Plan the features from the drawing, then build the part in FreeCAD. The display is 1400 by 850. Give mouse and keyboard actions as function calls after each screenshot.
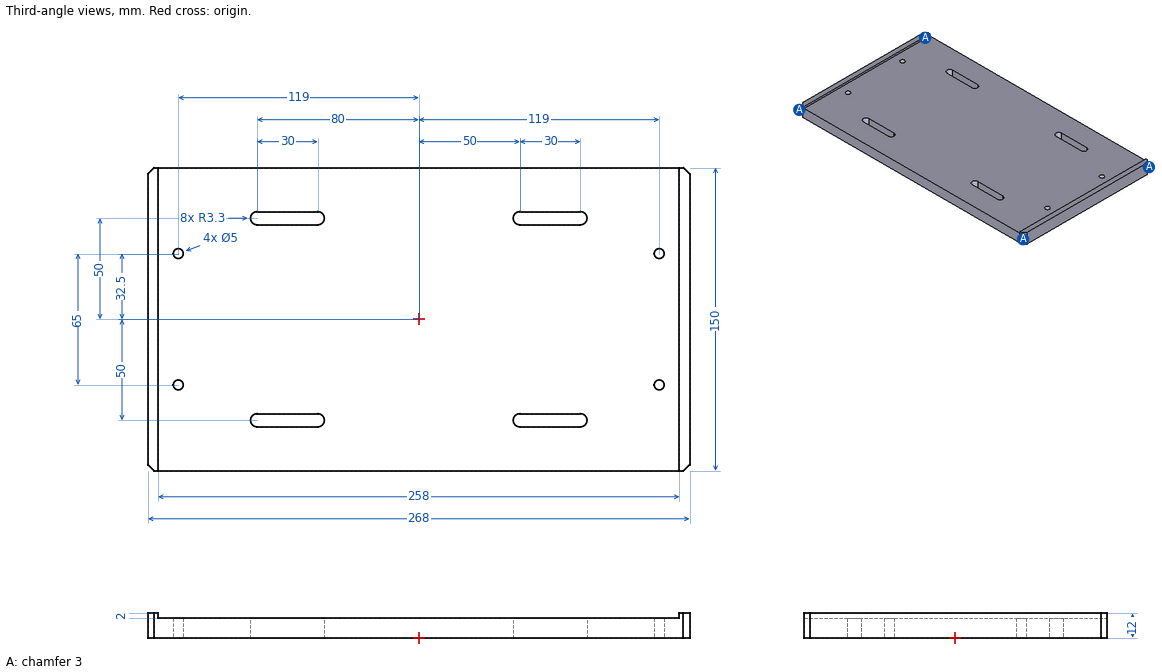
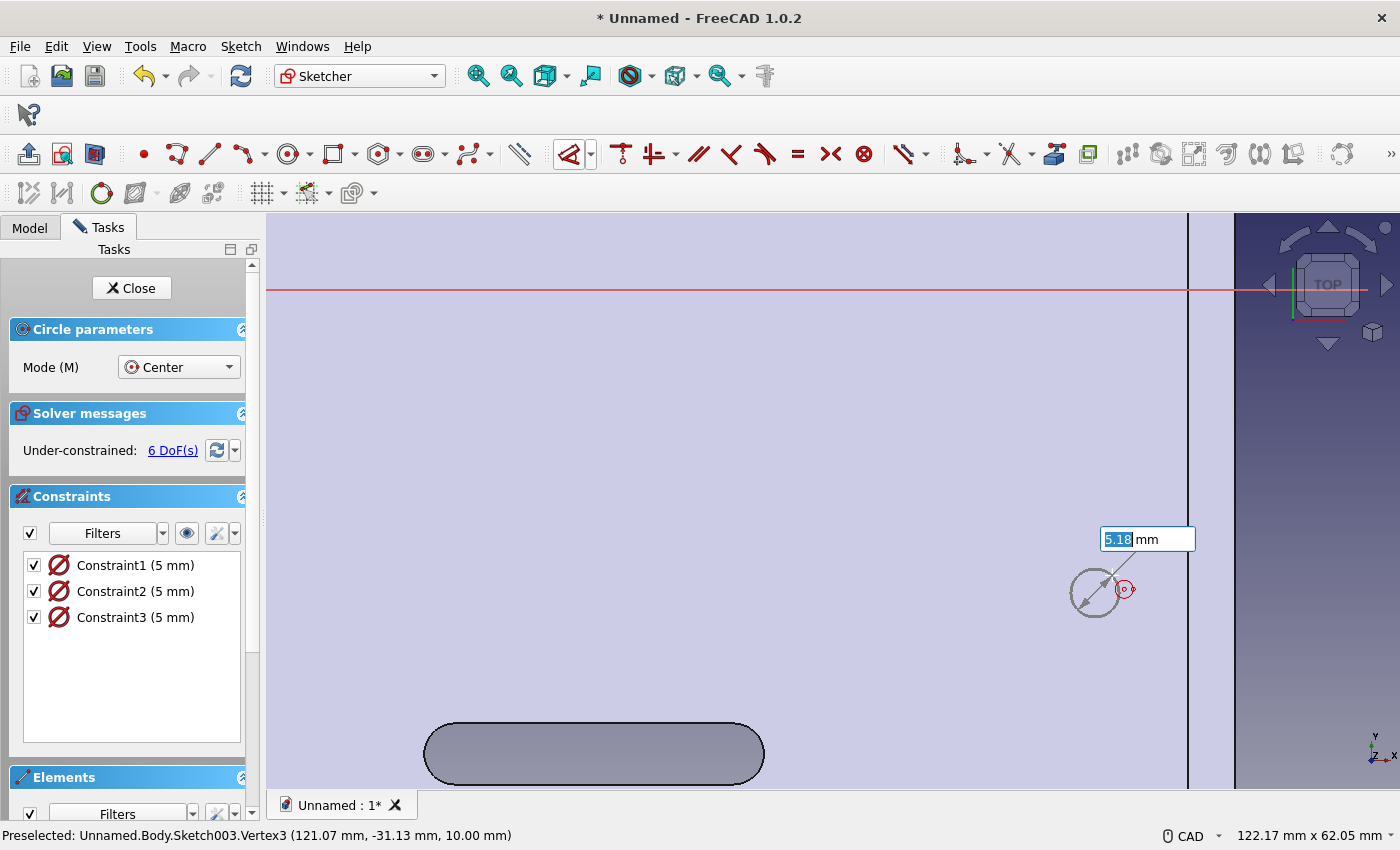
text(5)
key(Return)
key(Escape)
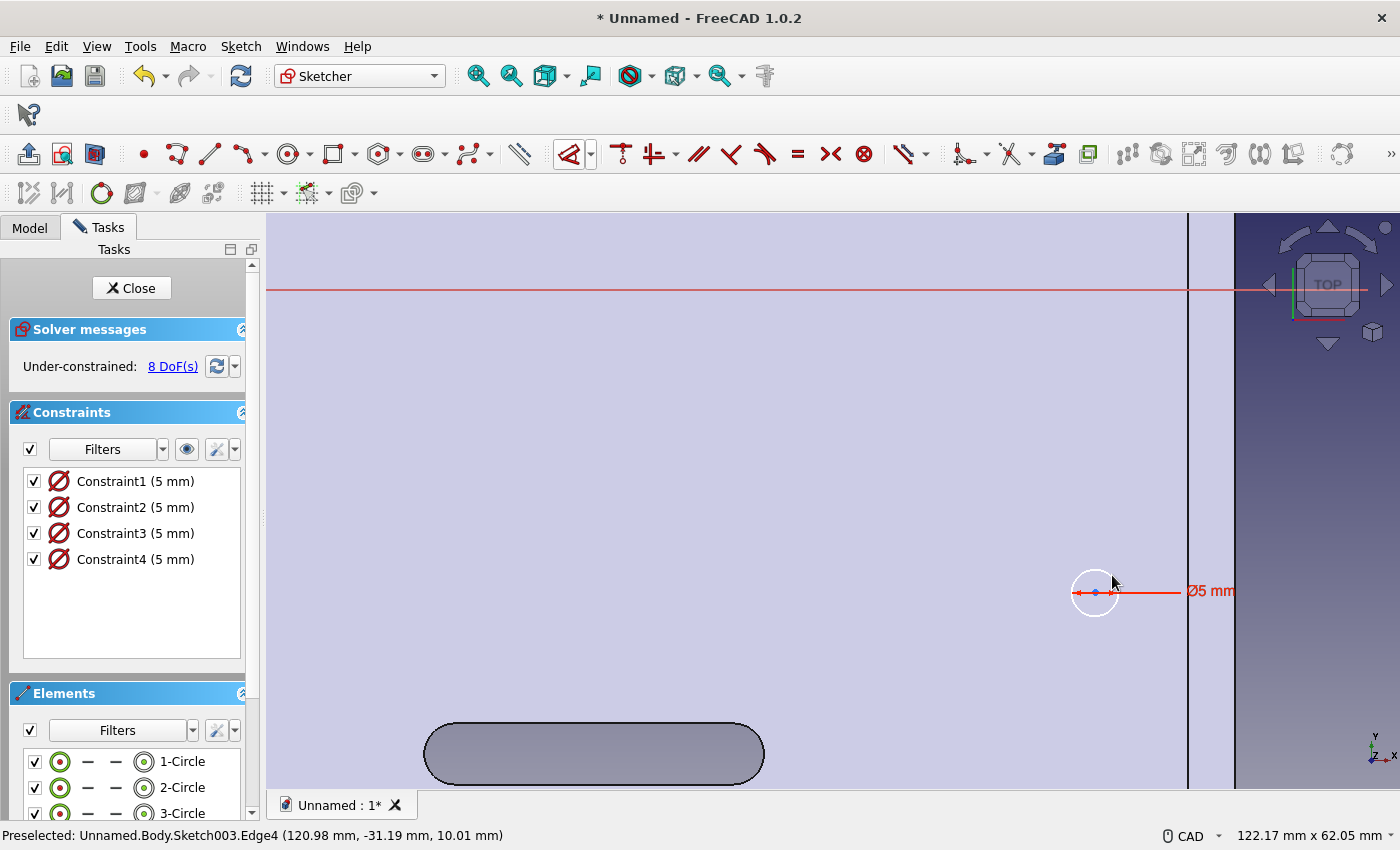
scroll(1098, 592, down, 6)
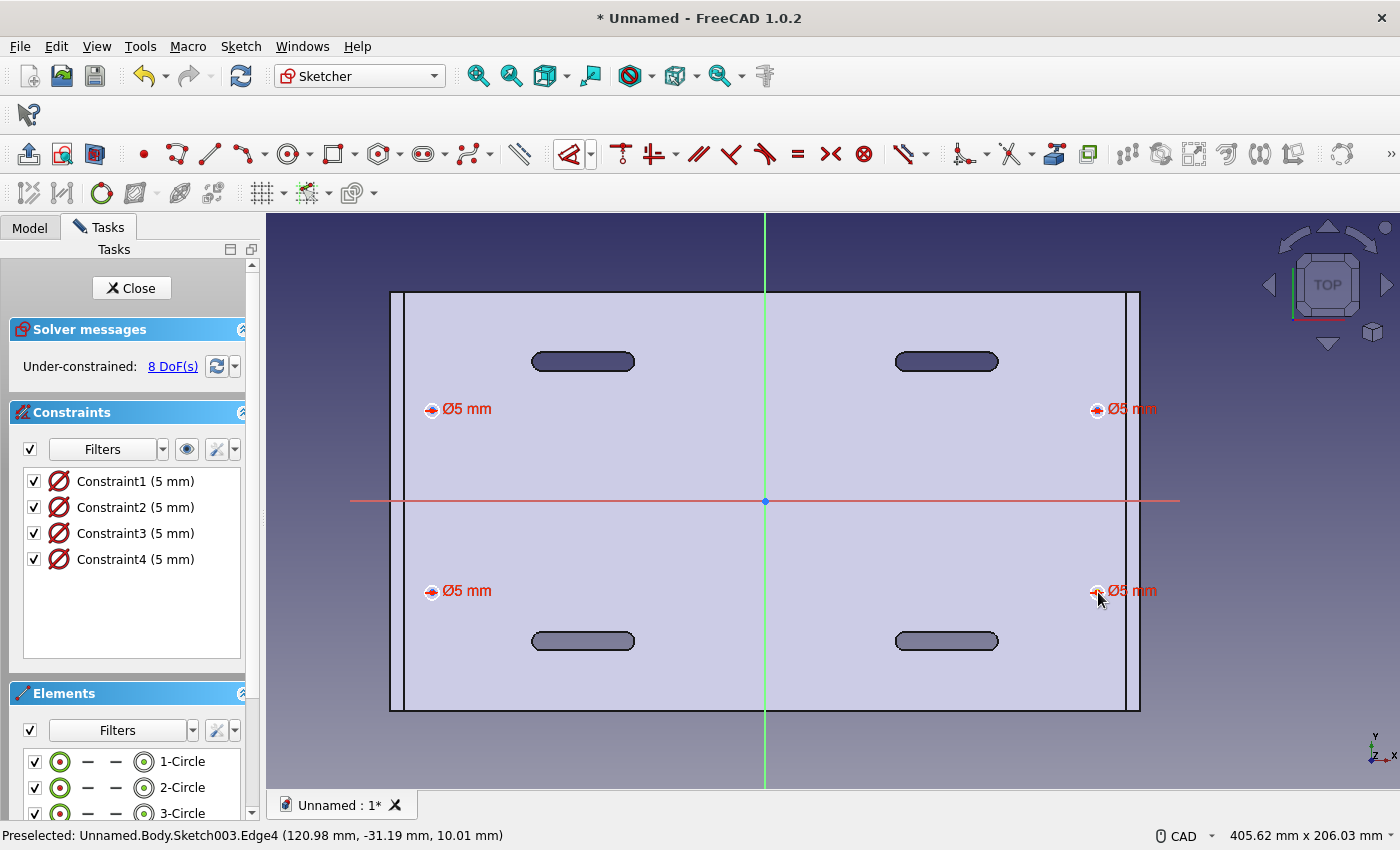
click(432, 411)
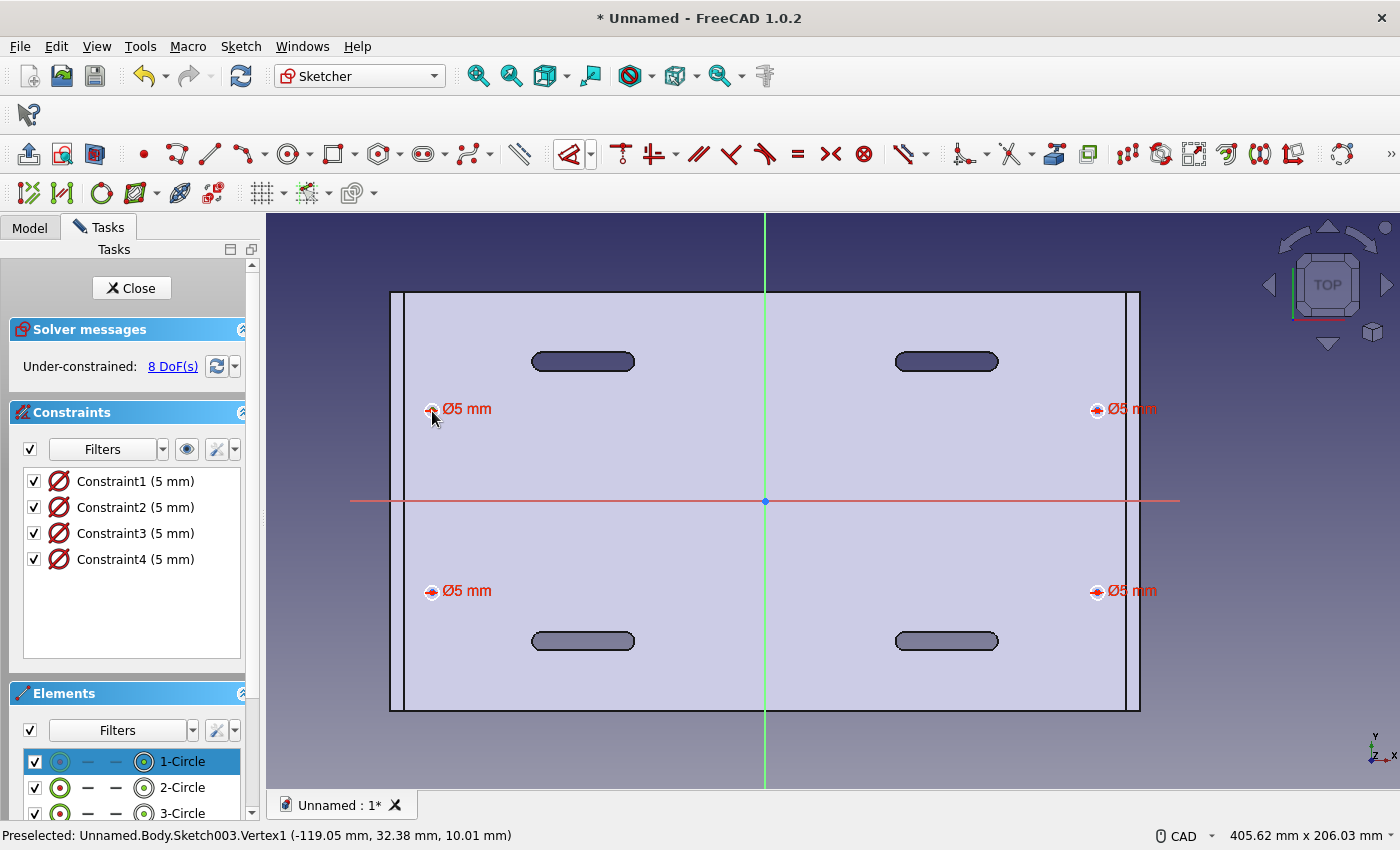
click(432, 593)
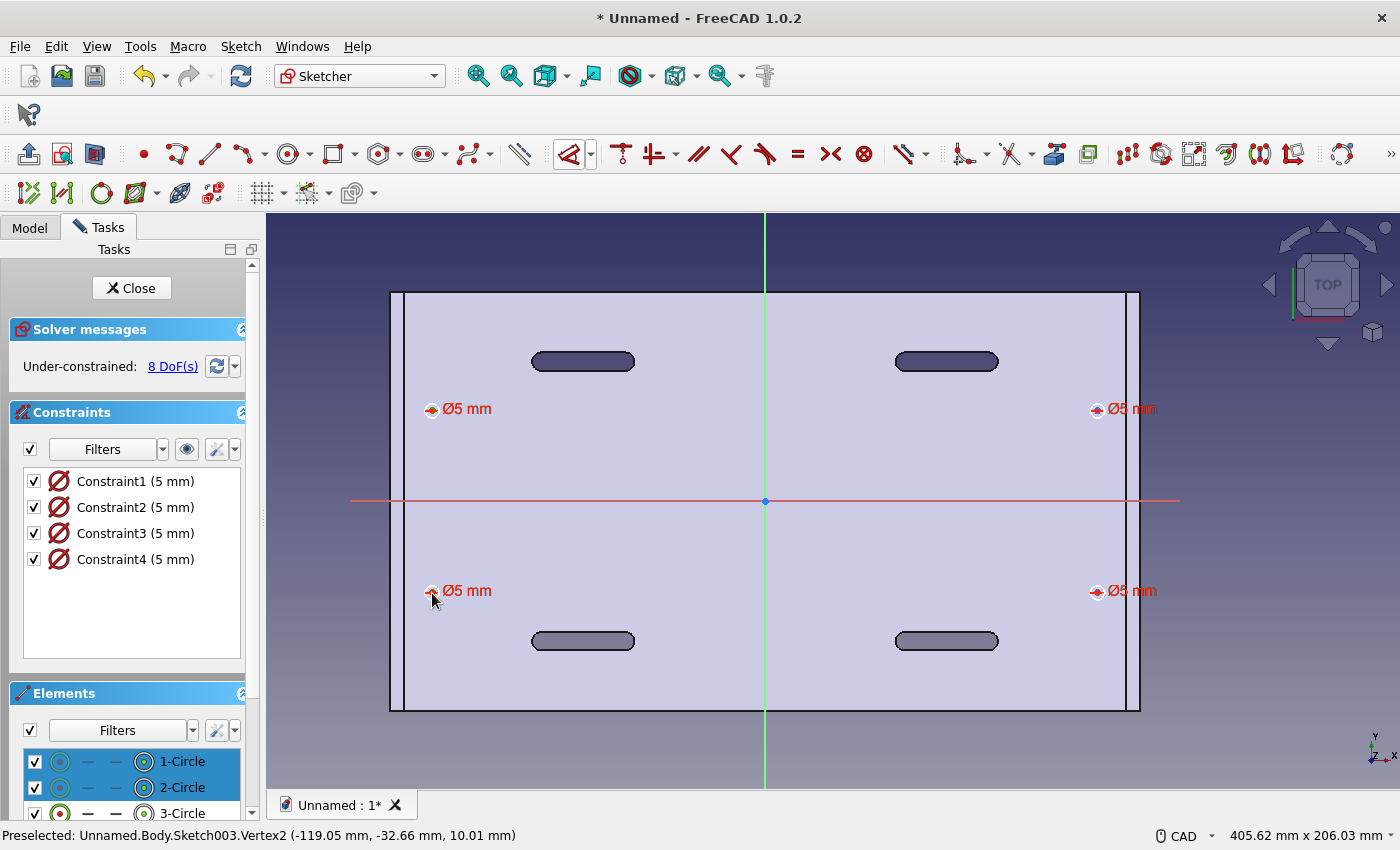
click(676, 154)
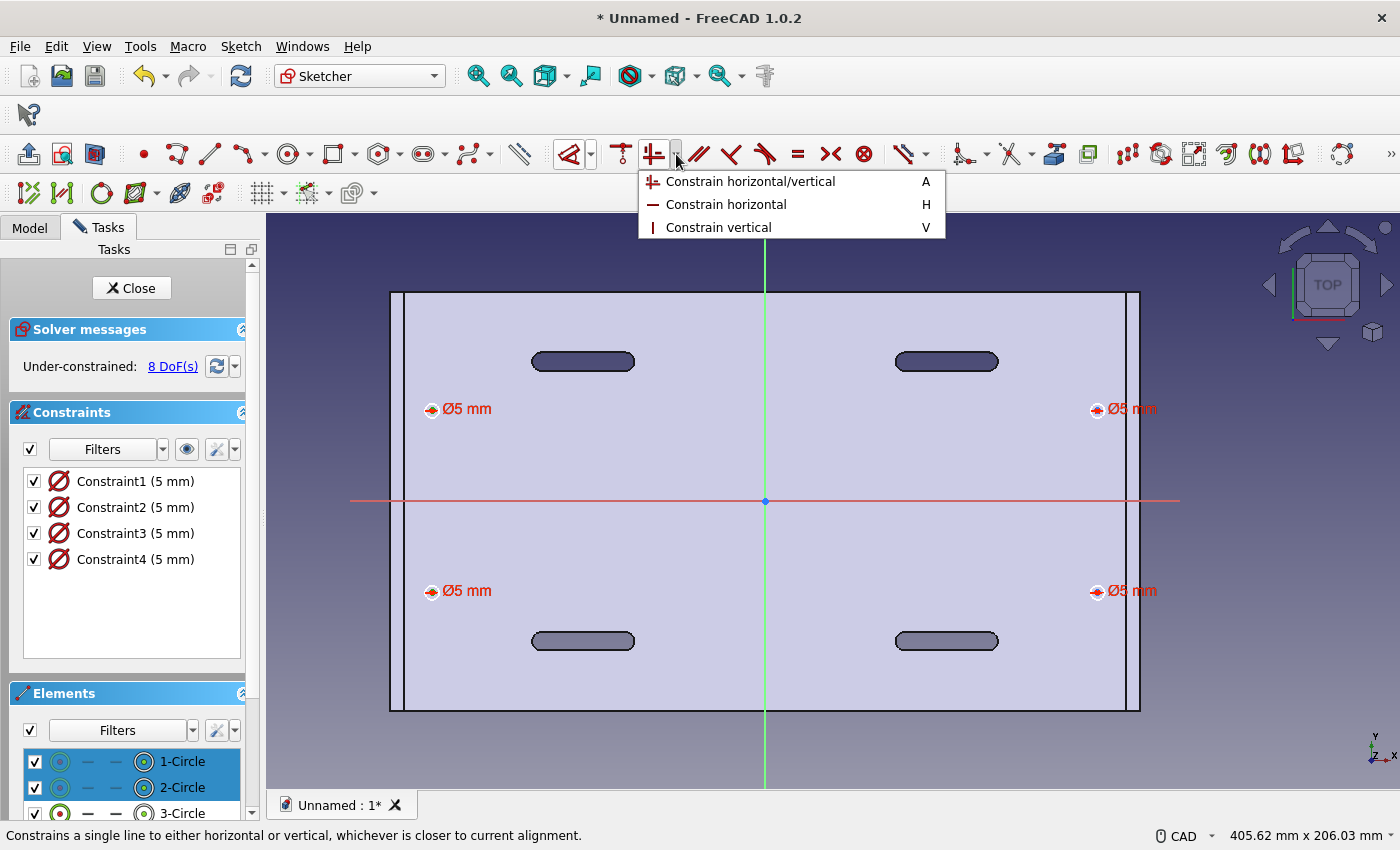
click(792, 228)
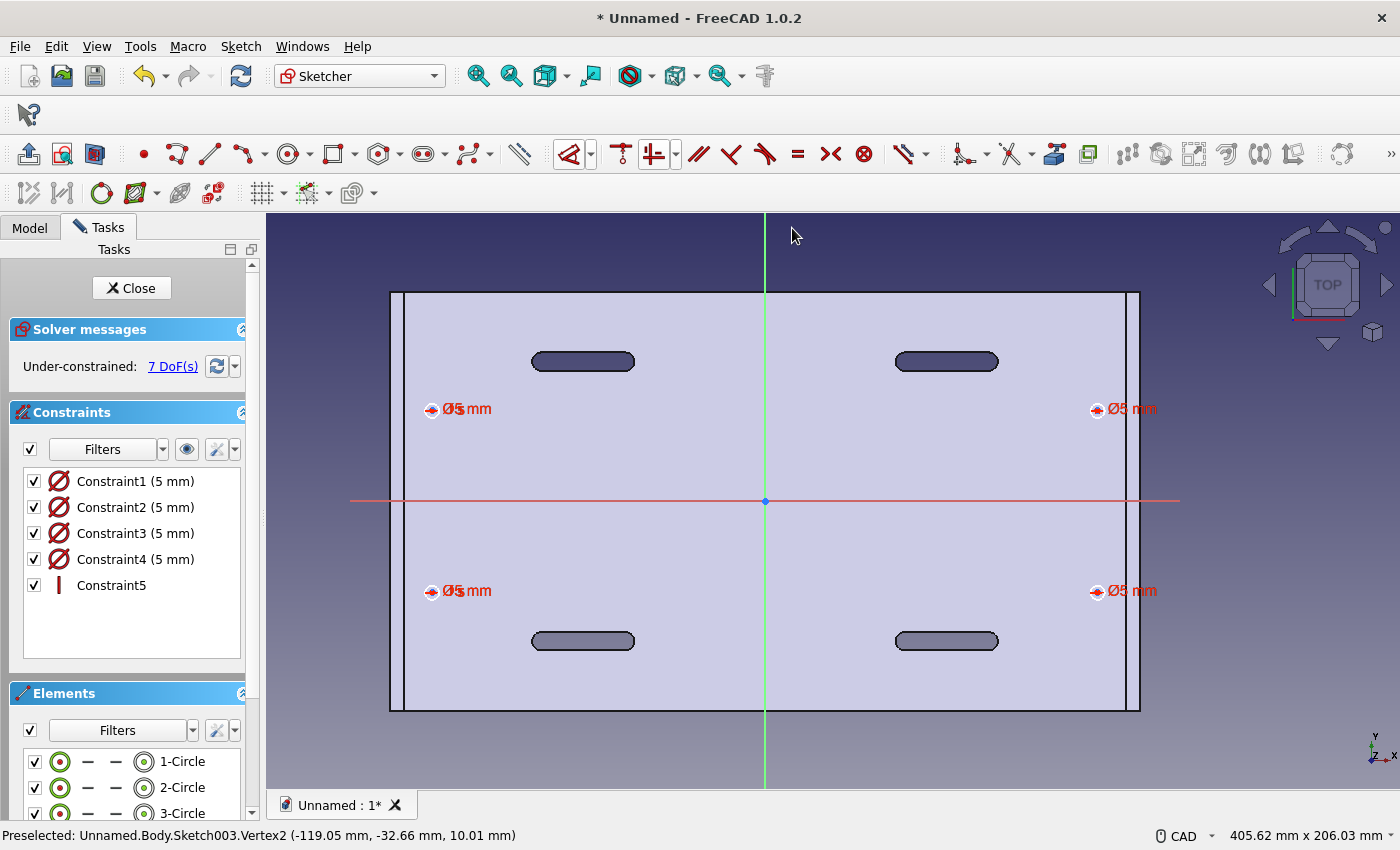
click(432, 411)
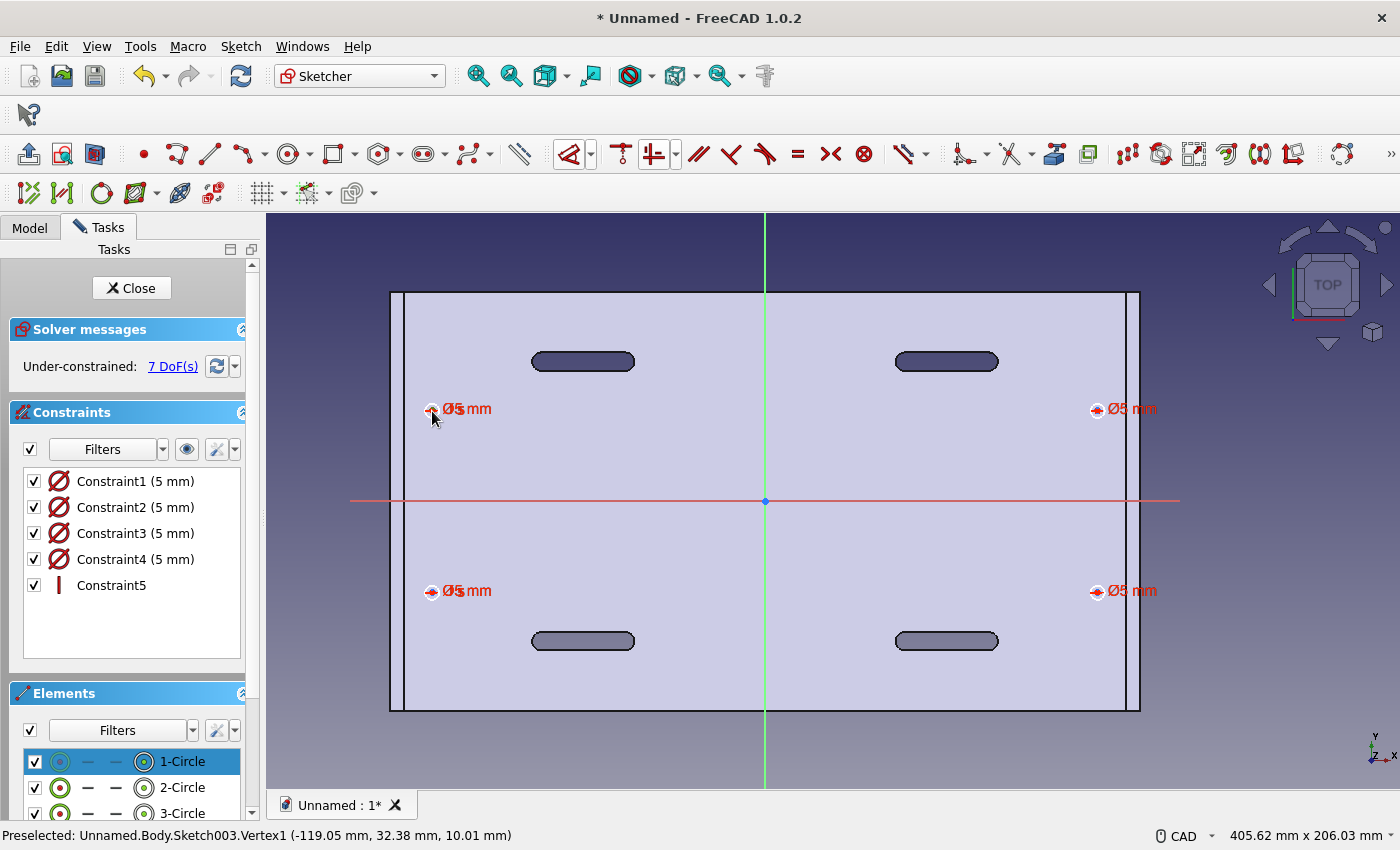
click(1098, 411)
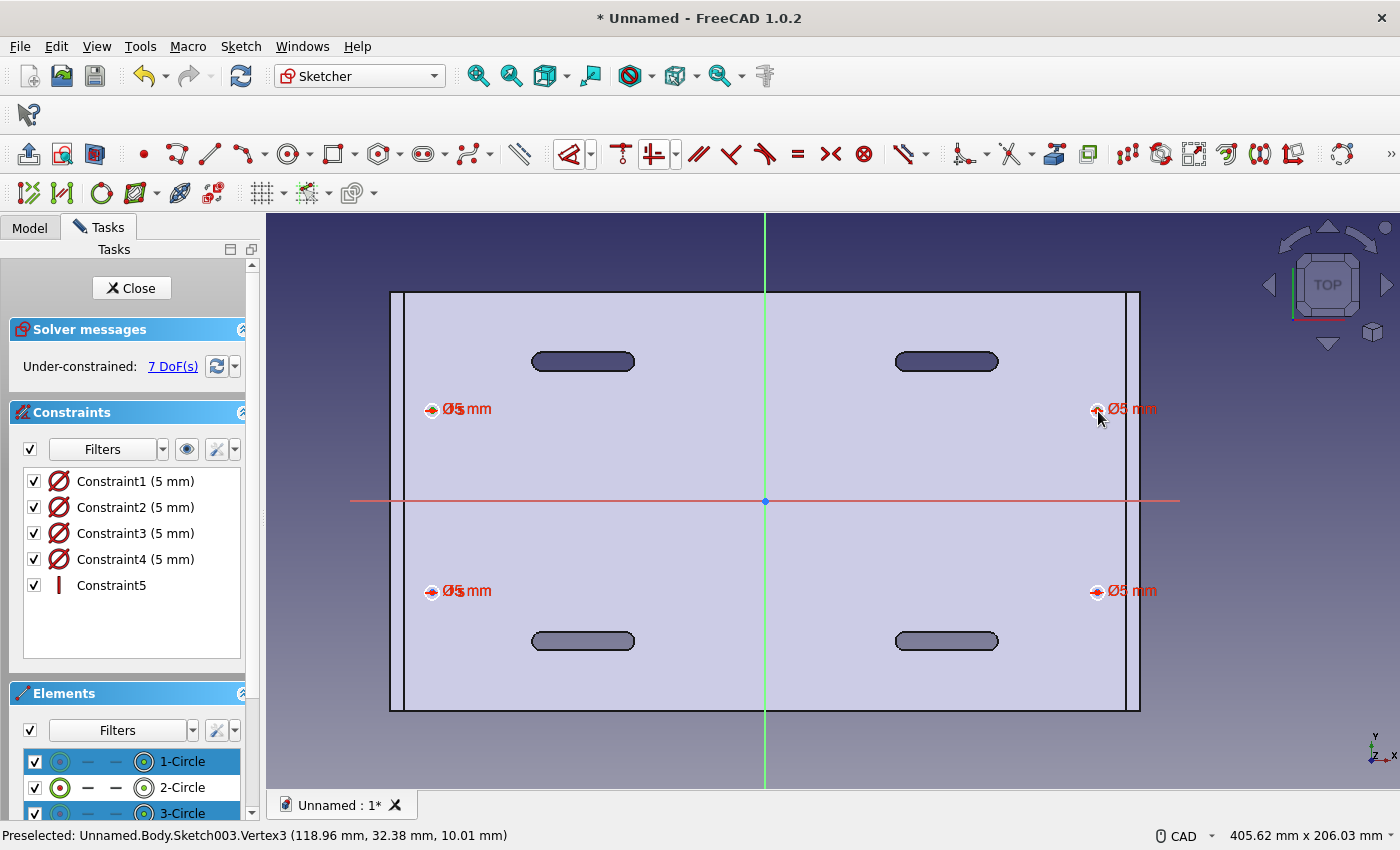
click(676, 154)